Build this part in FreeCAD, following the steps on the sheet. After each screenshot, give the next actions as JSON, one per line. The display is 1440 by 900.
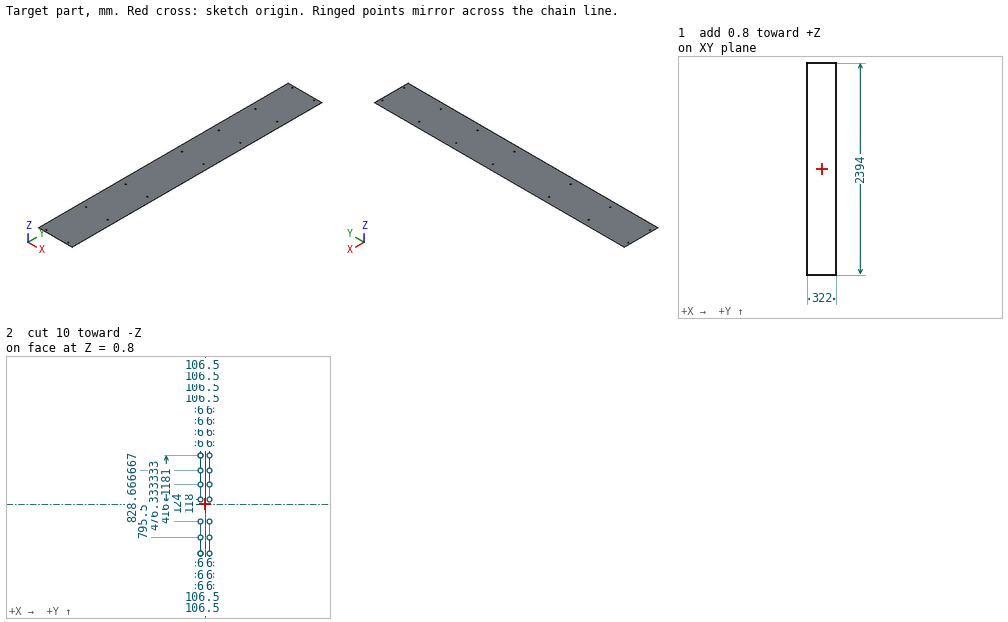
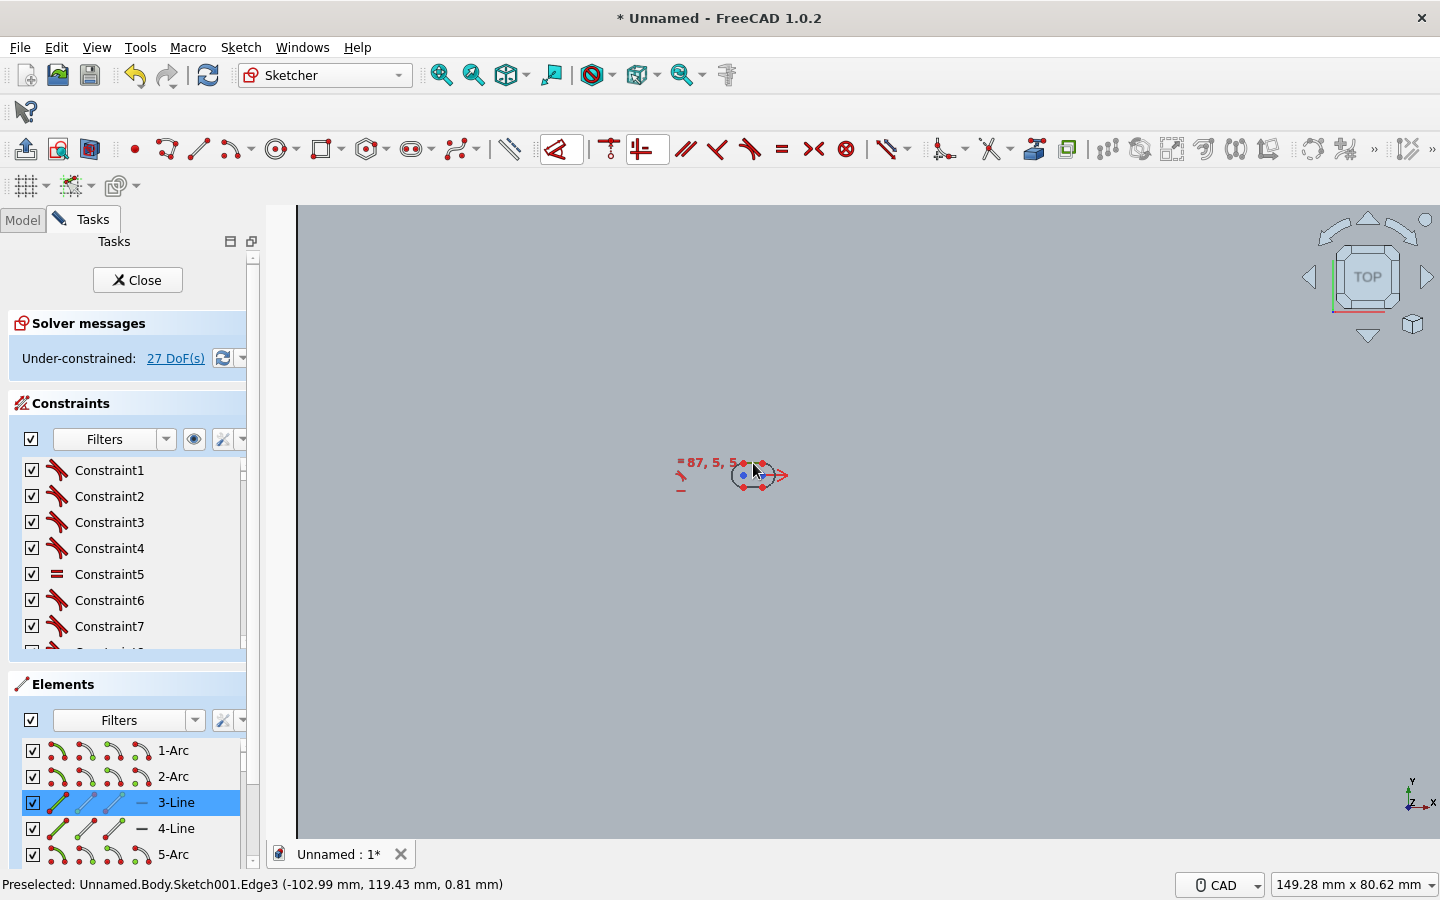
{"action": "left_click", "coordinate": [578, 150]}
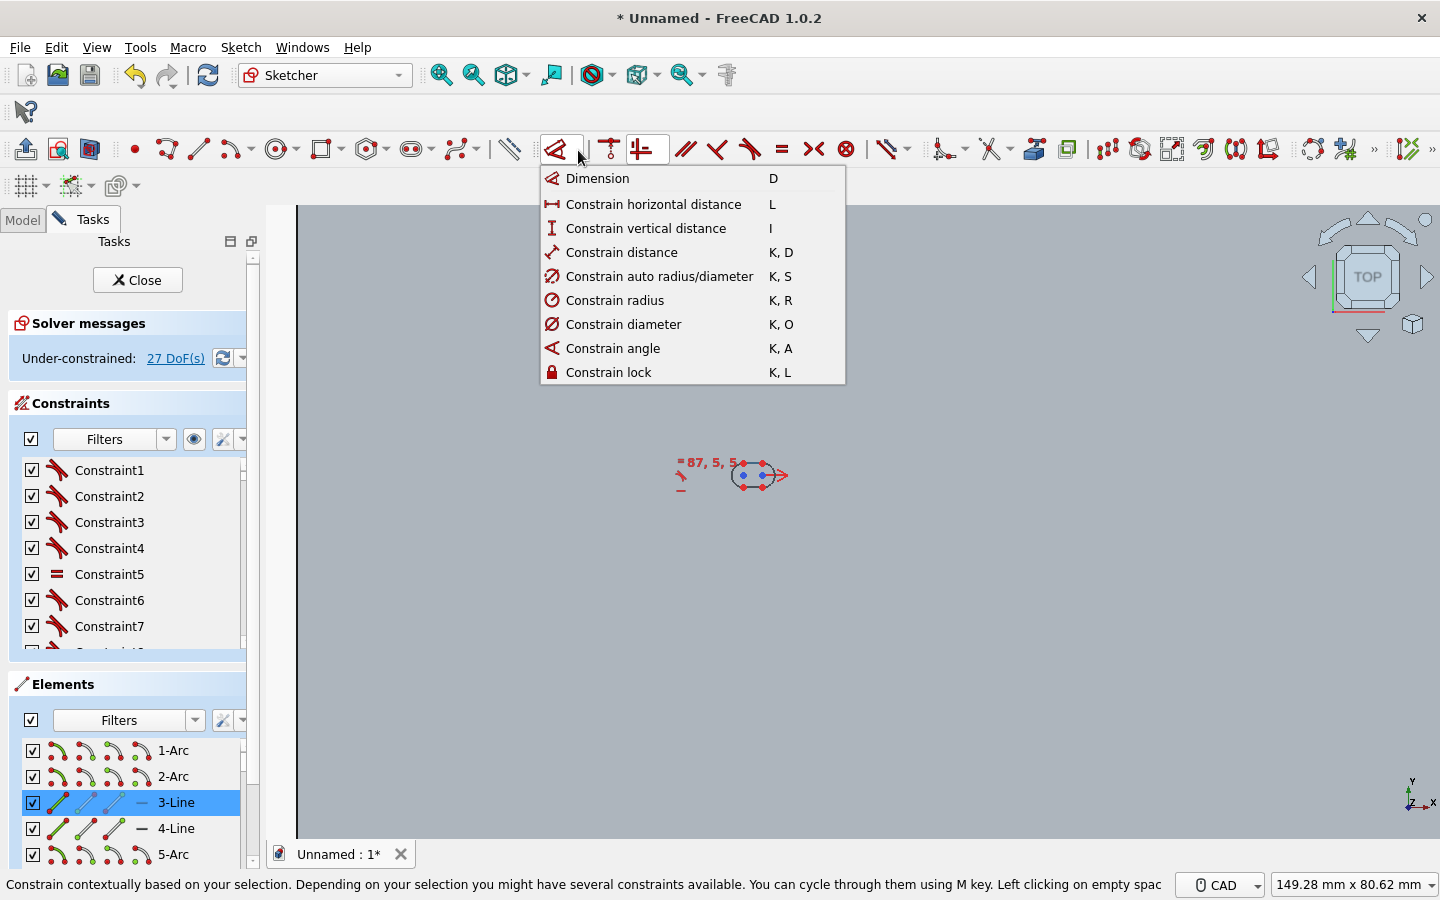
{"action": "left_click", "coordinate": [693, 204]}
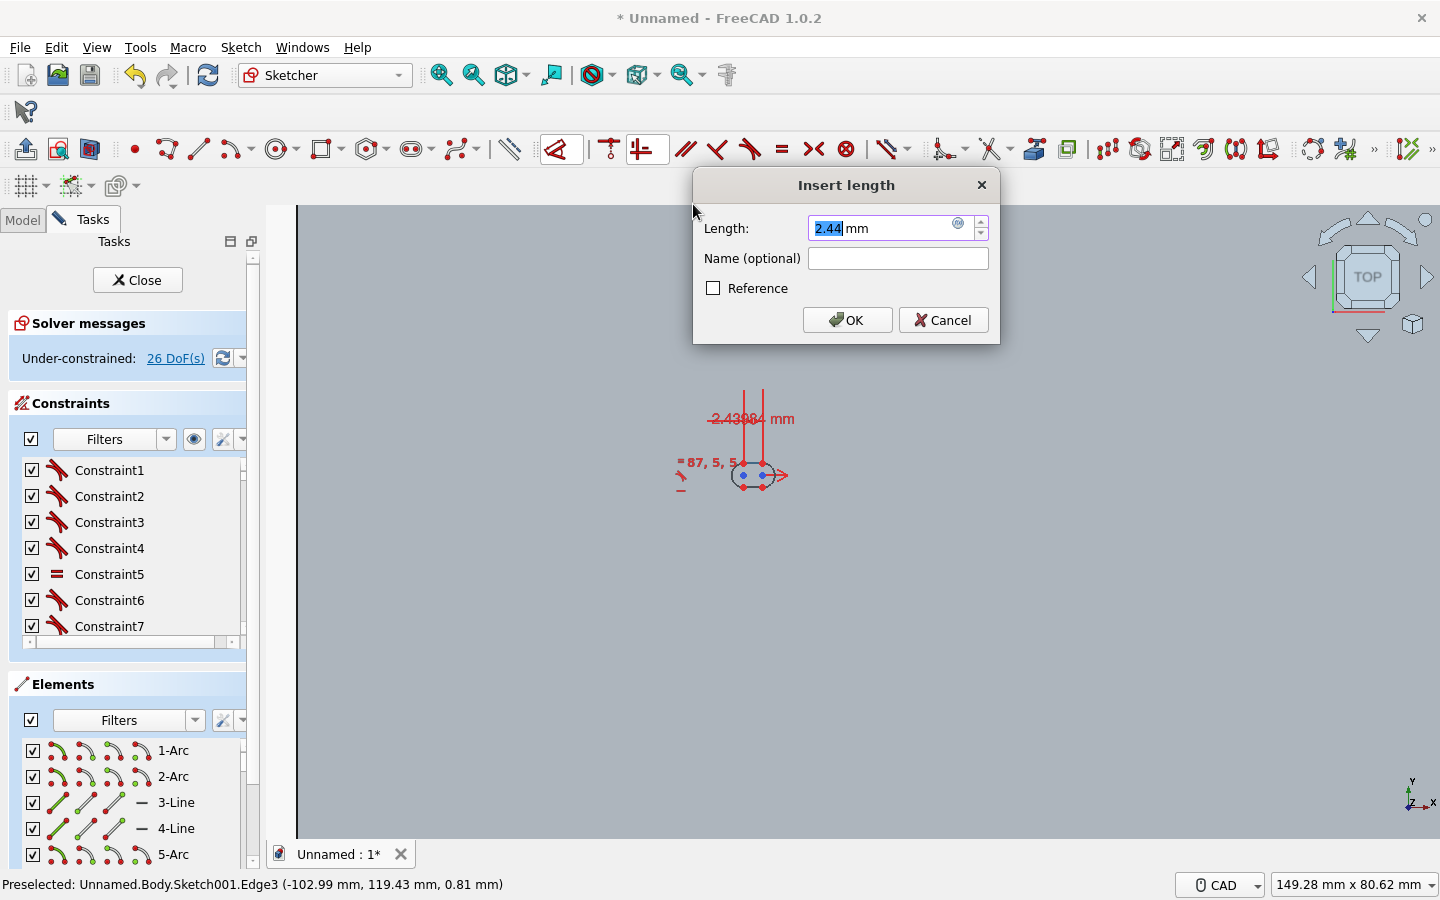
{"action": "type", "text": "6"}
{"action": "key", "text": "Return"}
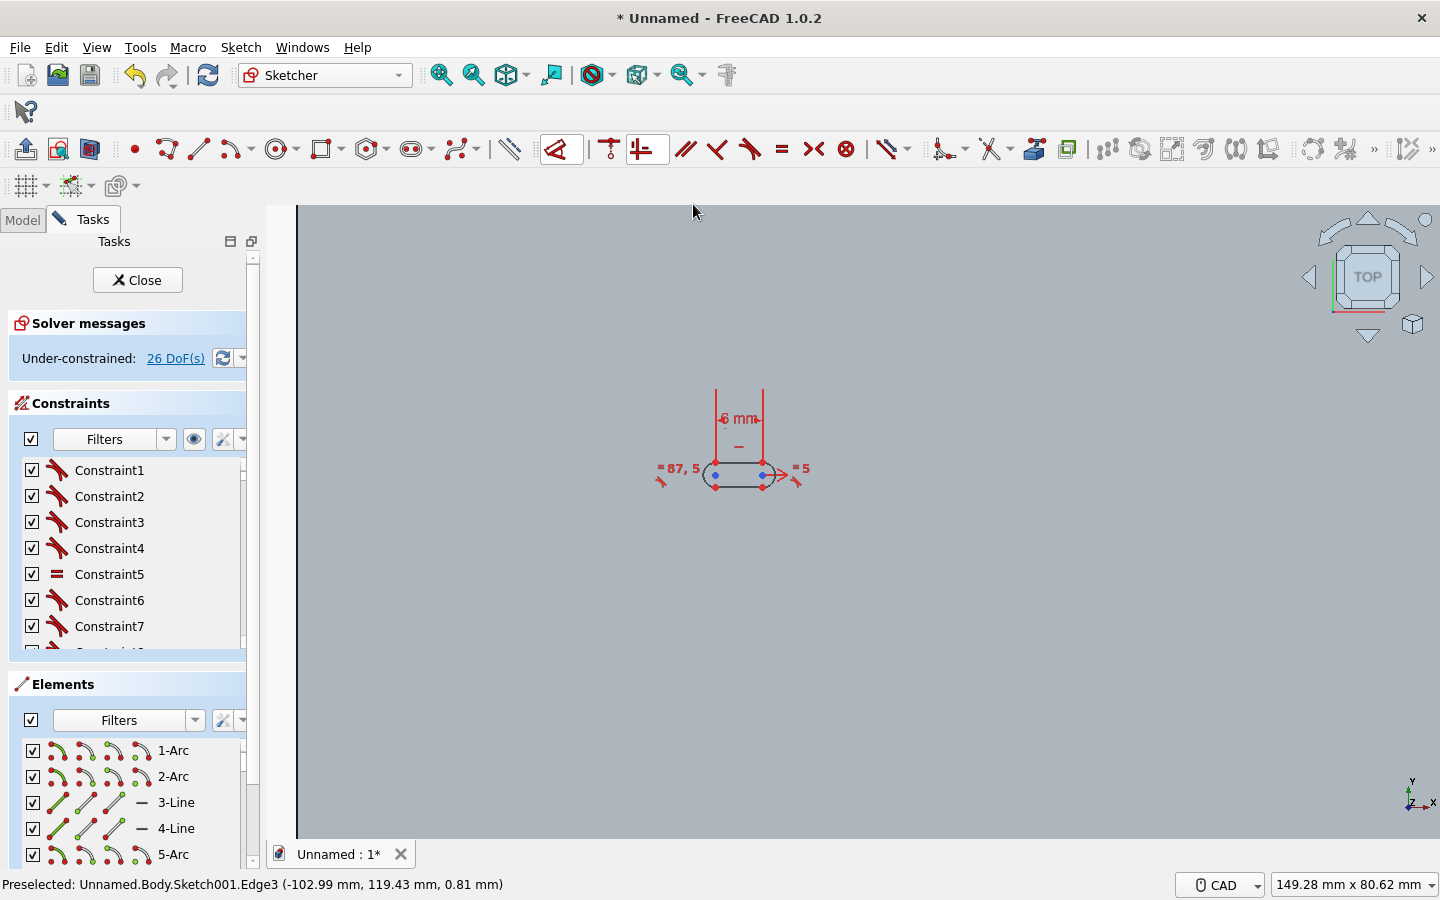
{"action": "scroll", "coordinate": [763, 497], "scroll_direction": "down", "scroll_amount": 18}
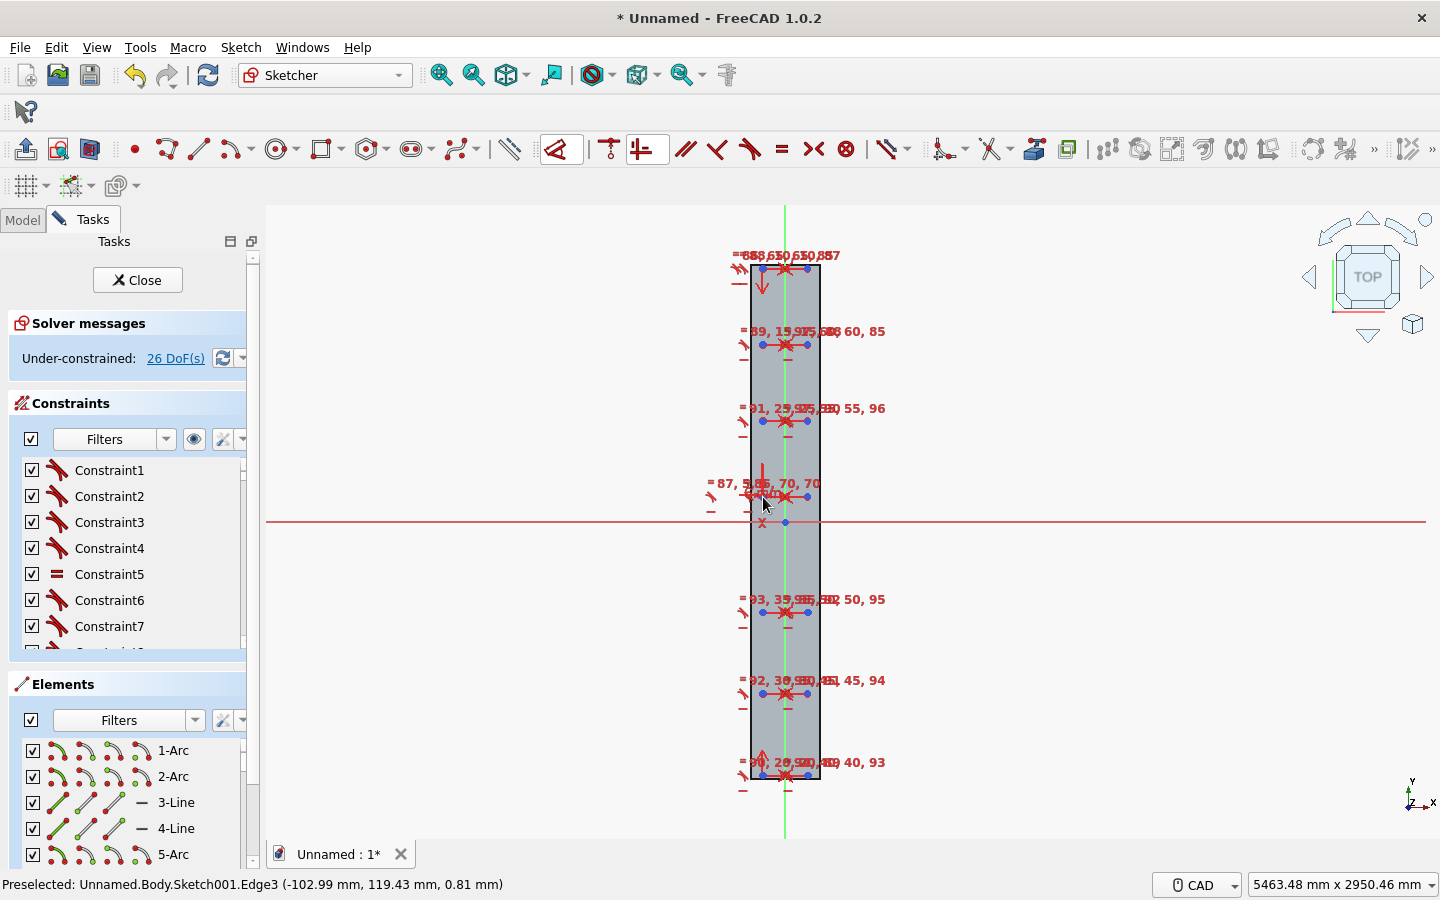
{"action": "scroll", "coordinate": [763, 268], "scroll_direction": "up", "scroll_amount": 18}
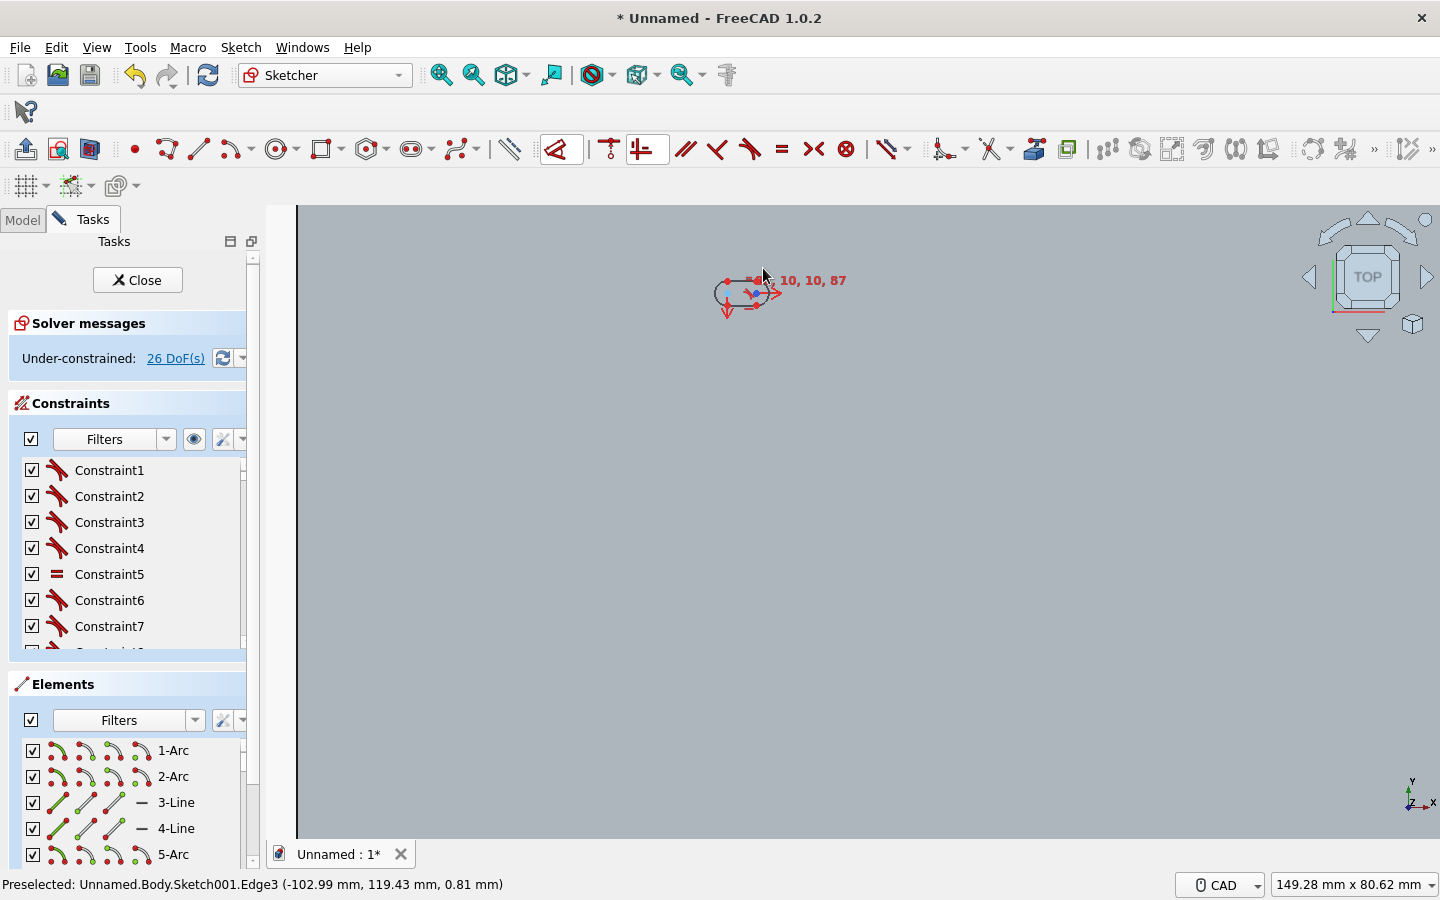
{"action": "left_click", "coordinate": [739, 281]}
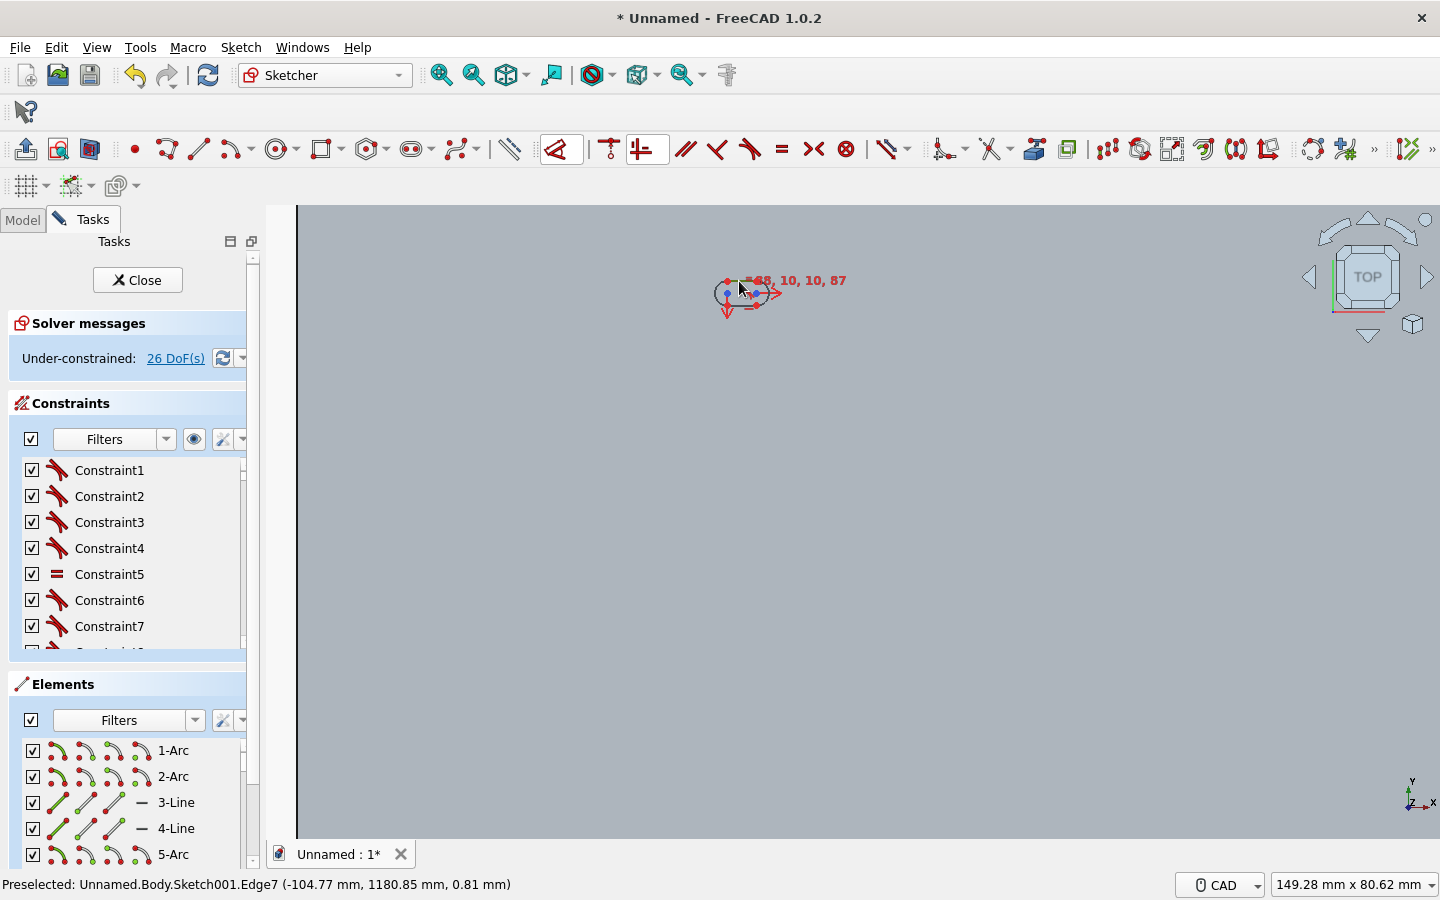
{"action": "left_click", "coordinate": [578, 150]}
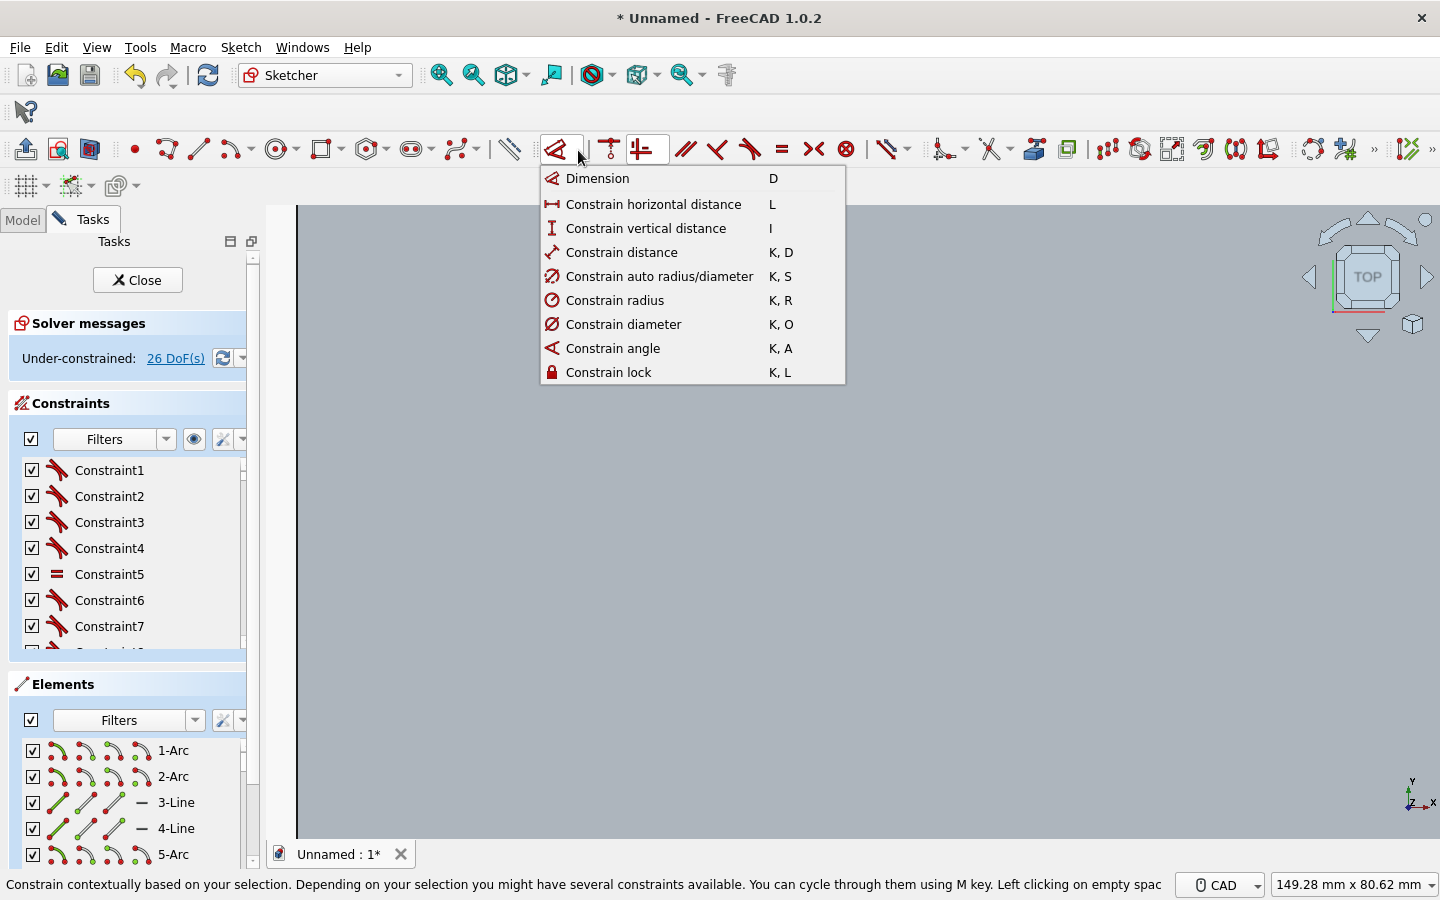
{"action": "left_click", "coordinate": [693, 204]}